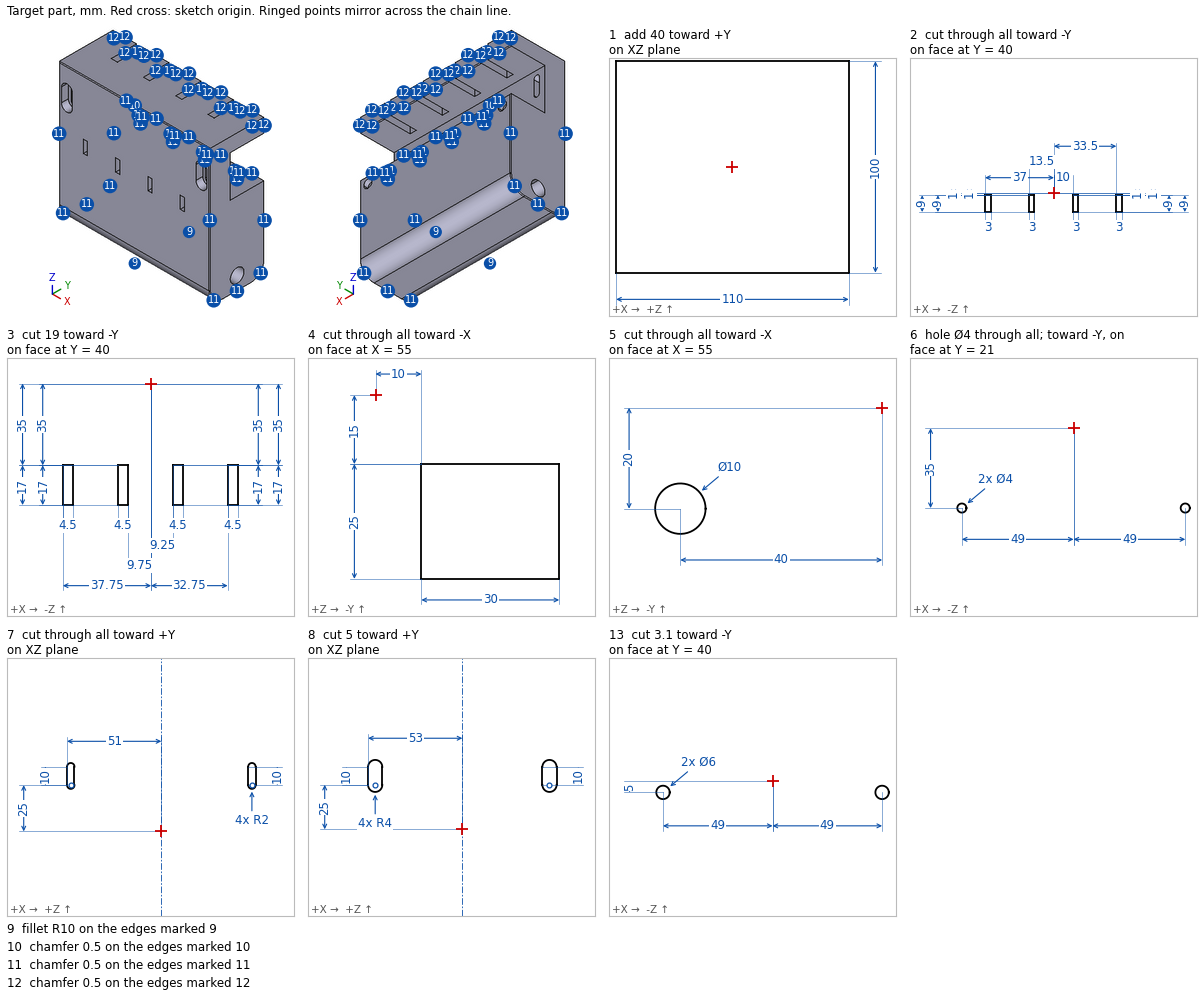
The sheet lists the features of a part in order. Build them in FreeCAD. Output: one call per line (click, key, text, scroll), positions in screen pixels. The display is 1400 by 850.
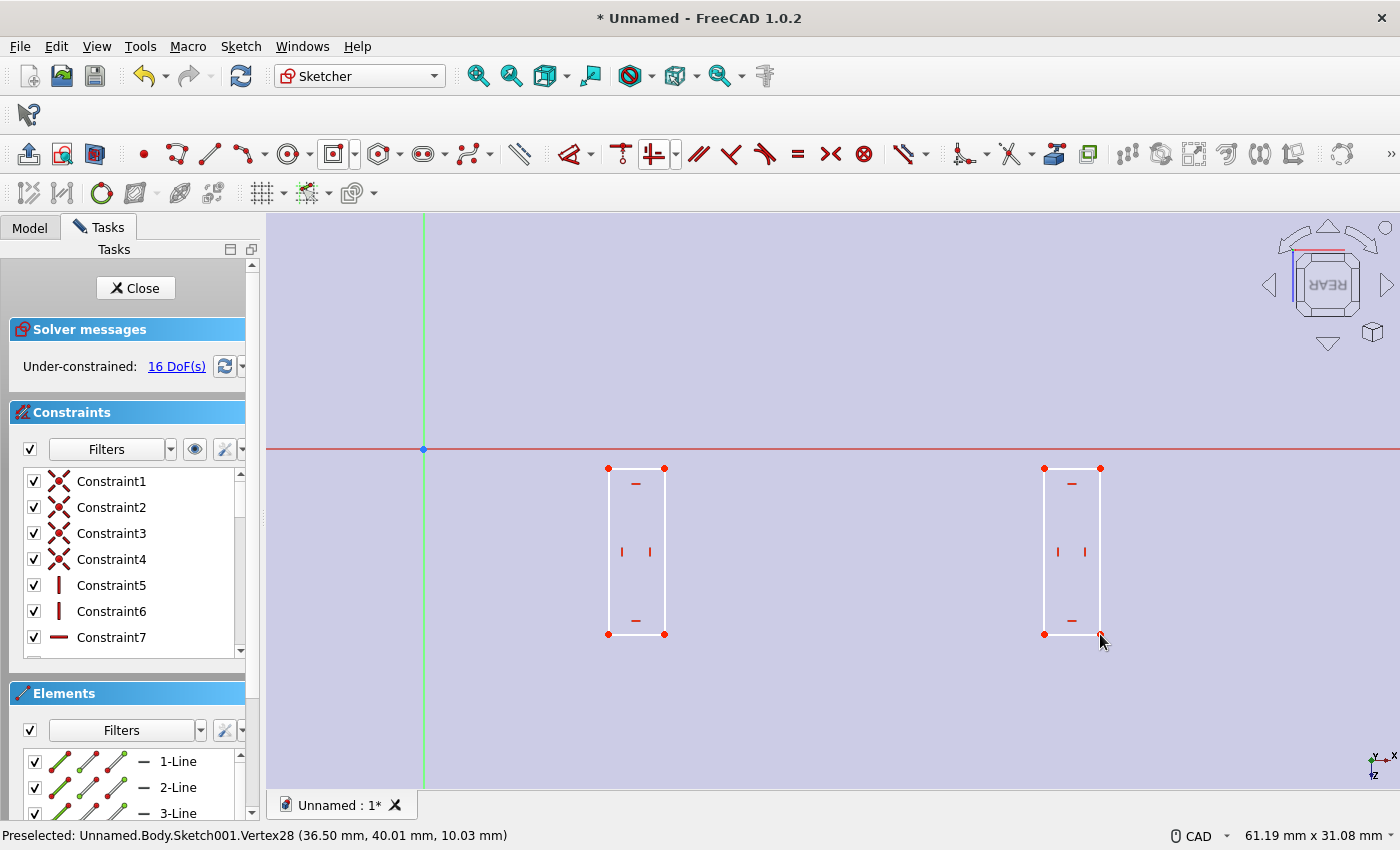
key(d)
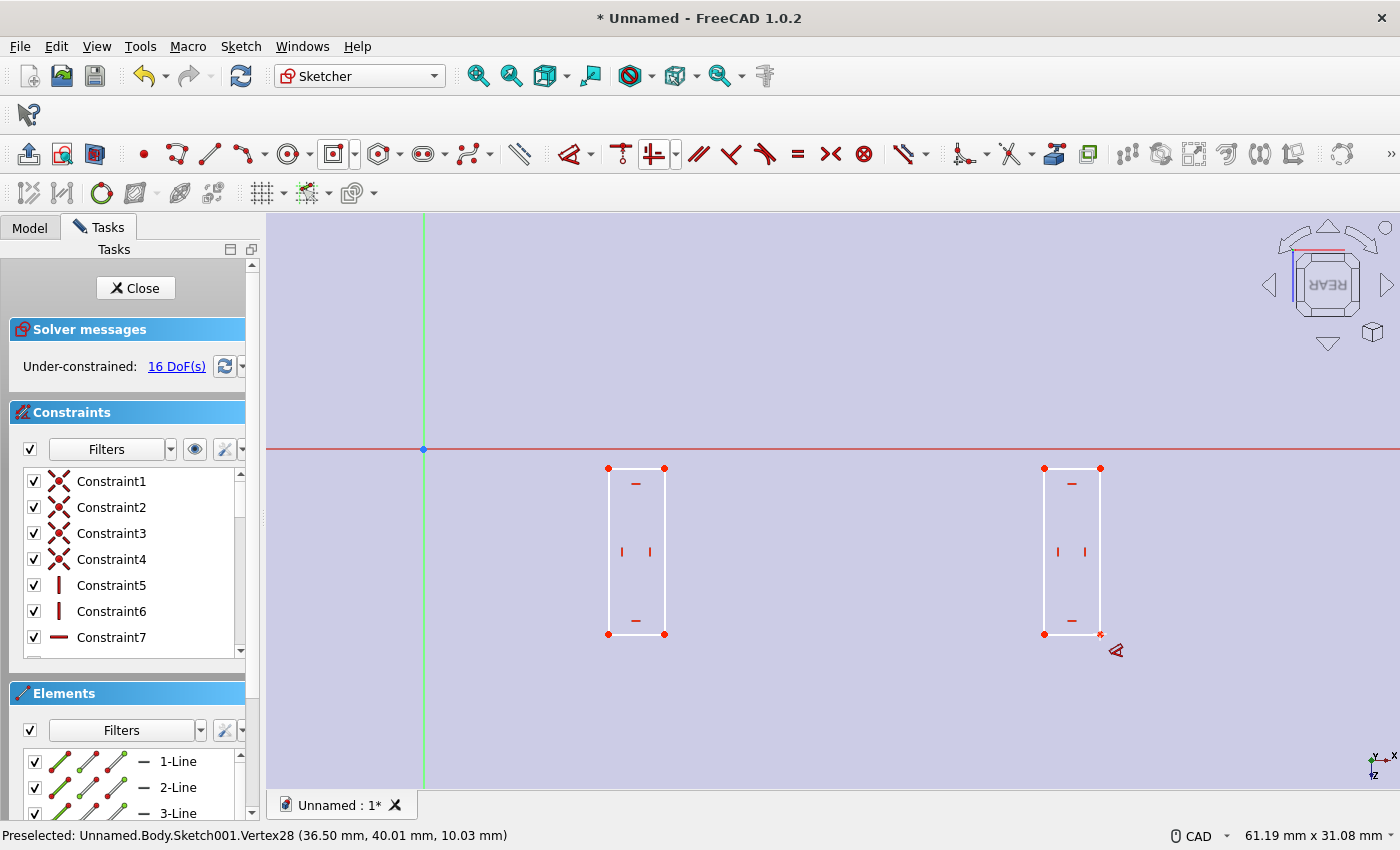
scroll(1046, 468, down, 4)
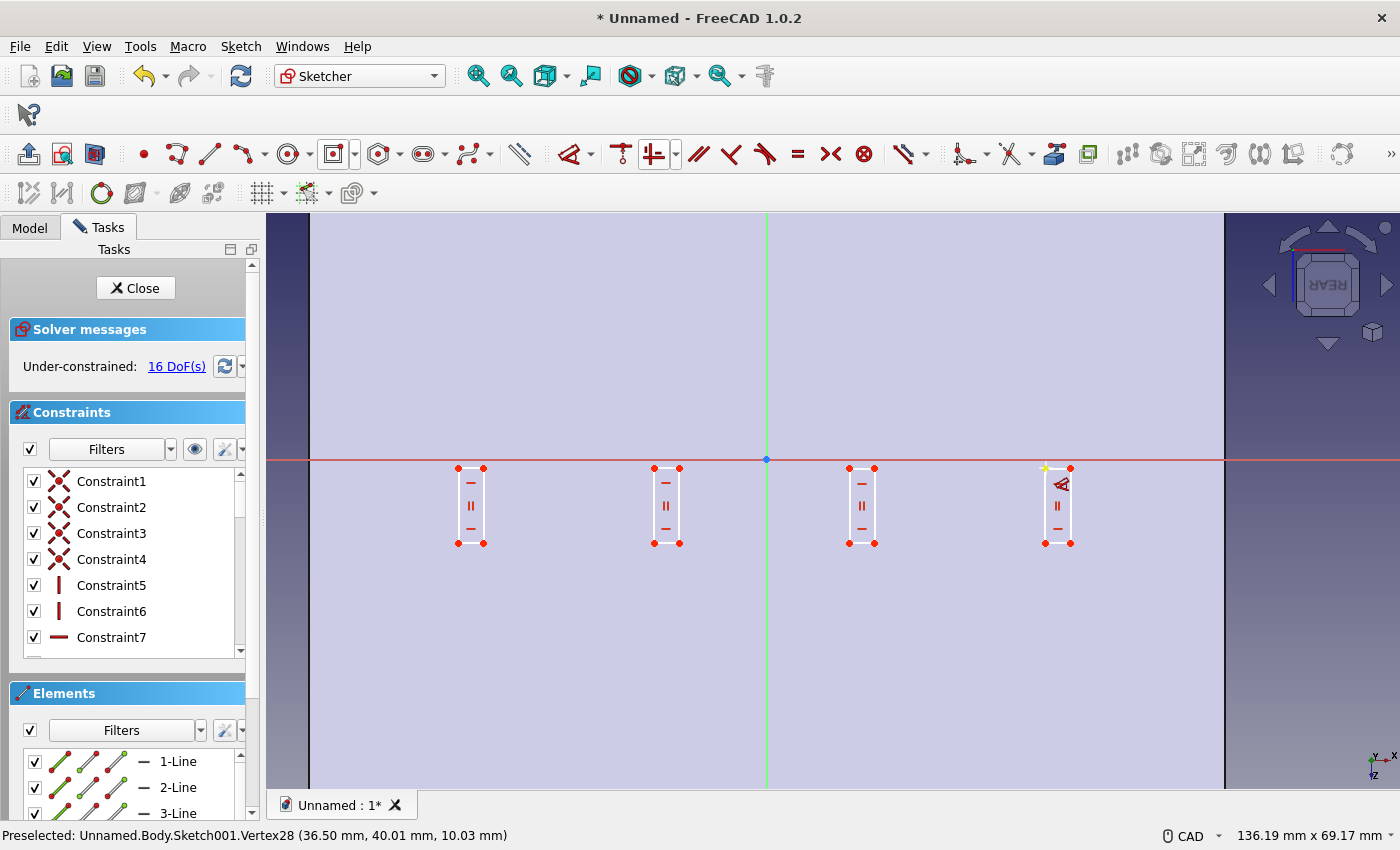
click(459, 491)
click(425, 506)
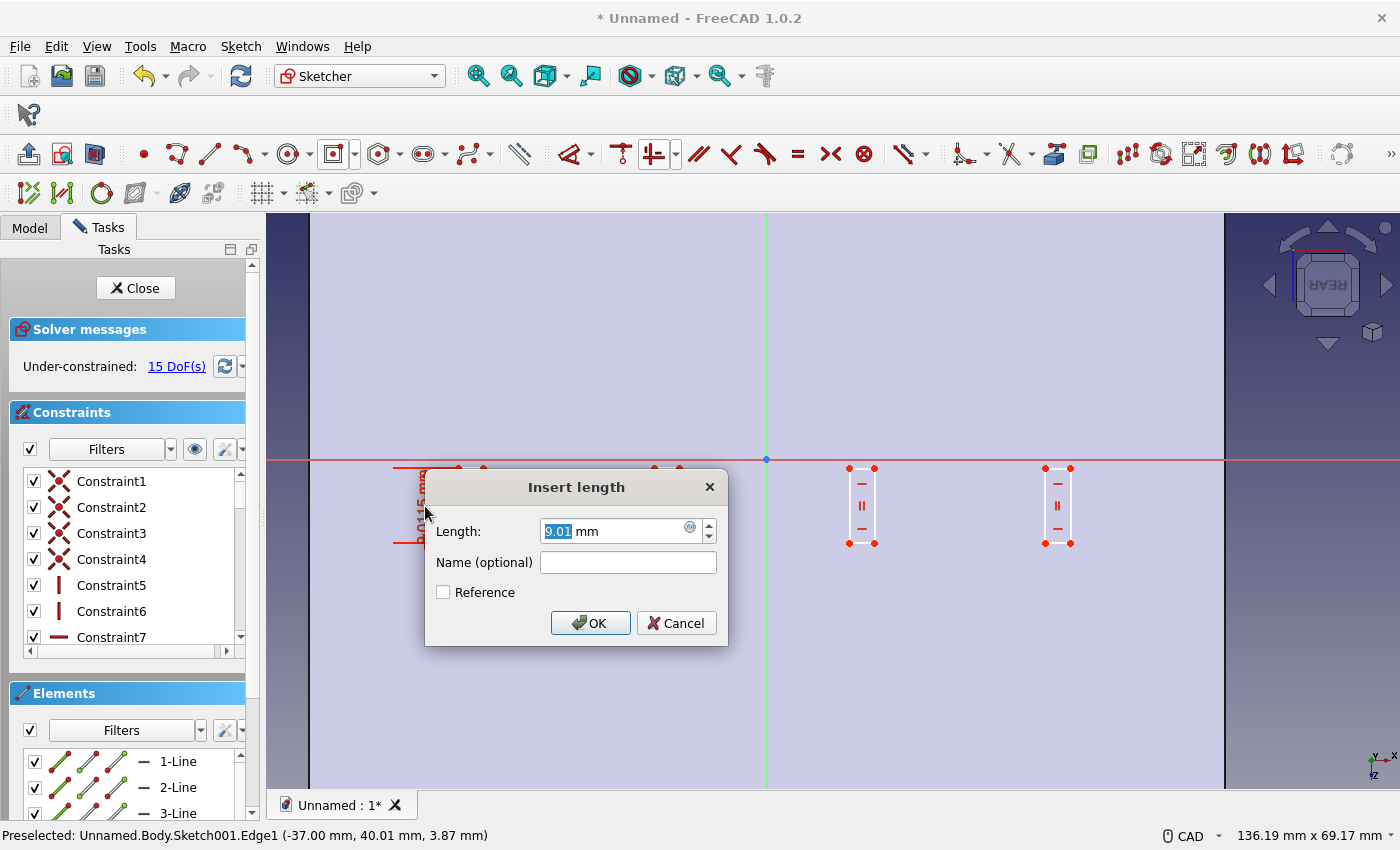
text(9)
key(Return)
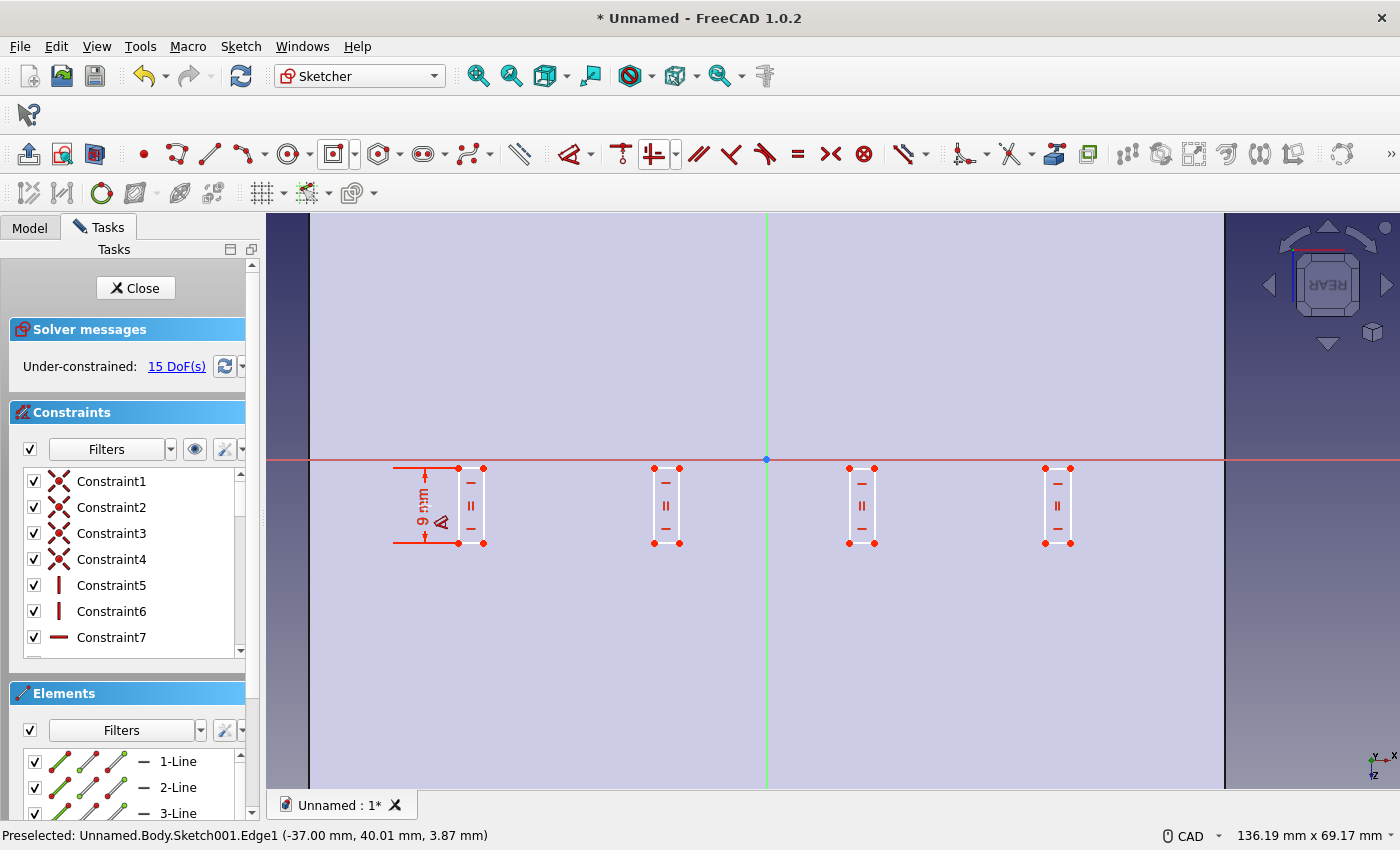
scroll(469, 543, up, 3)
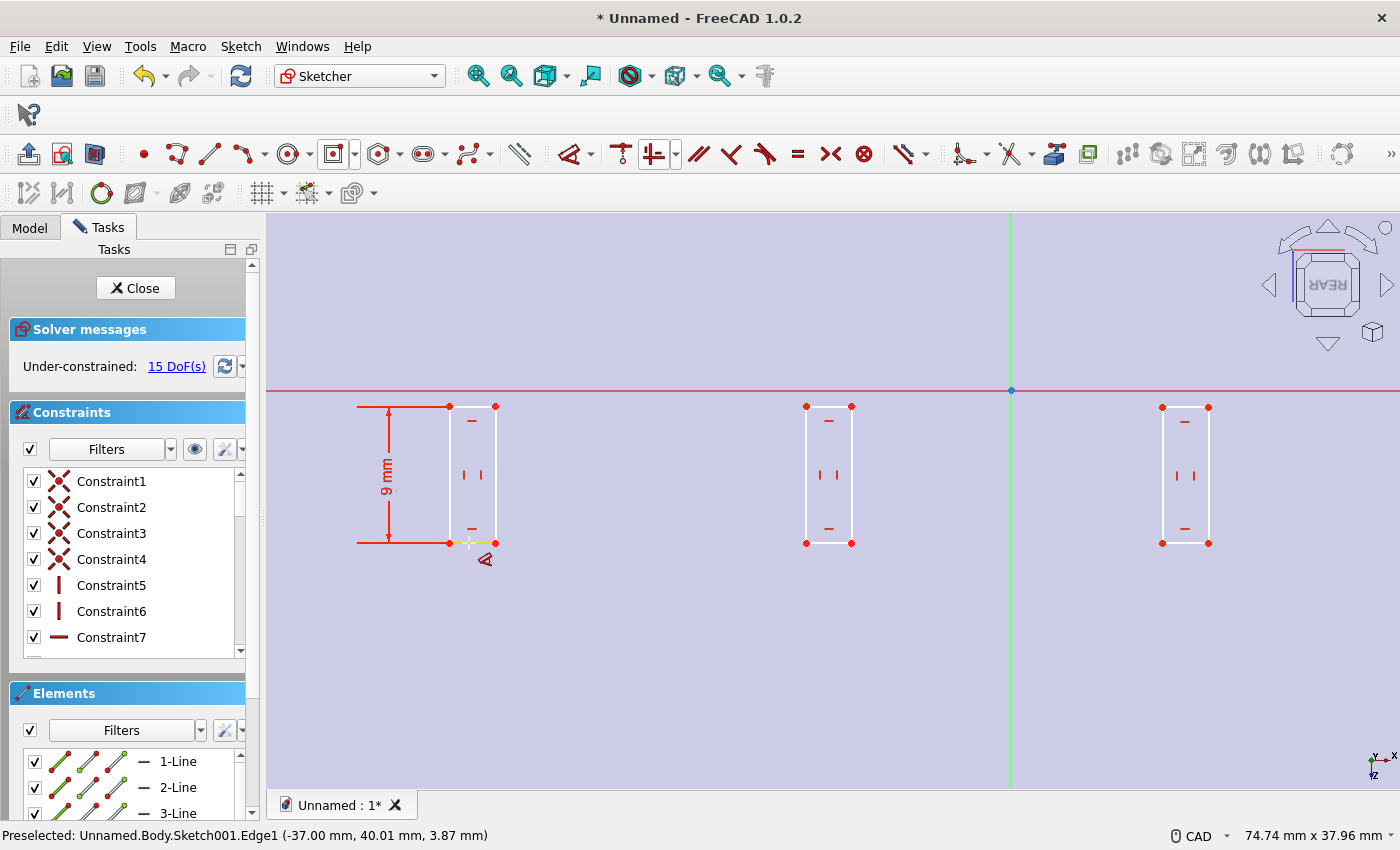
click(468, 543)
click(473, 577)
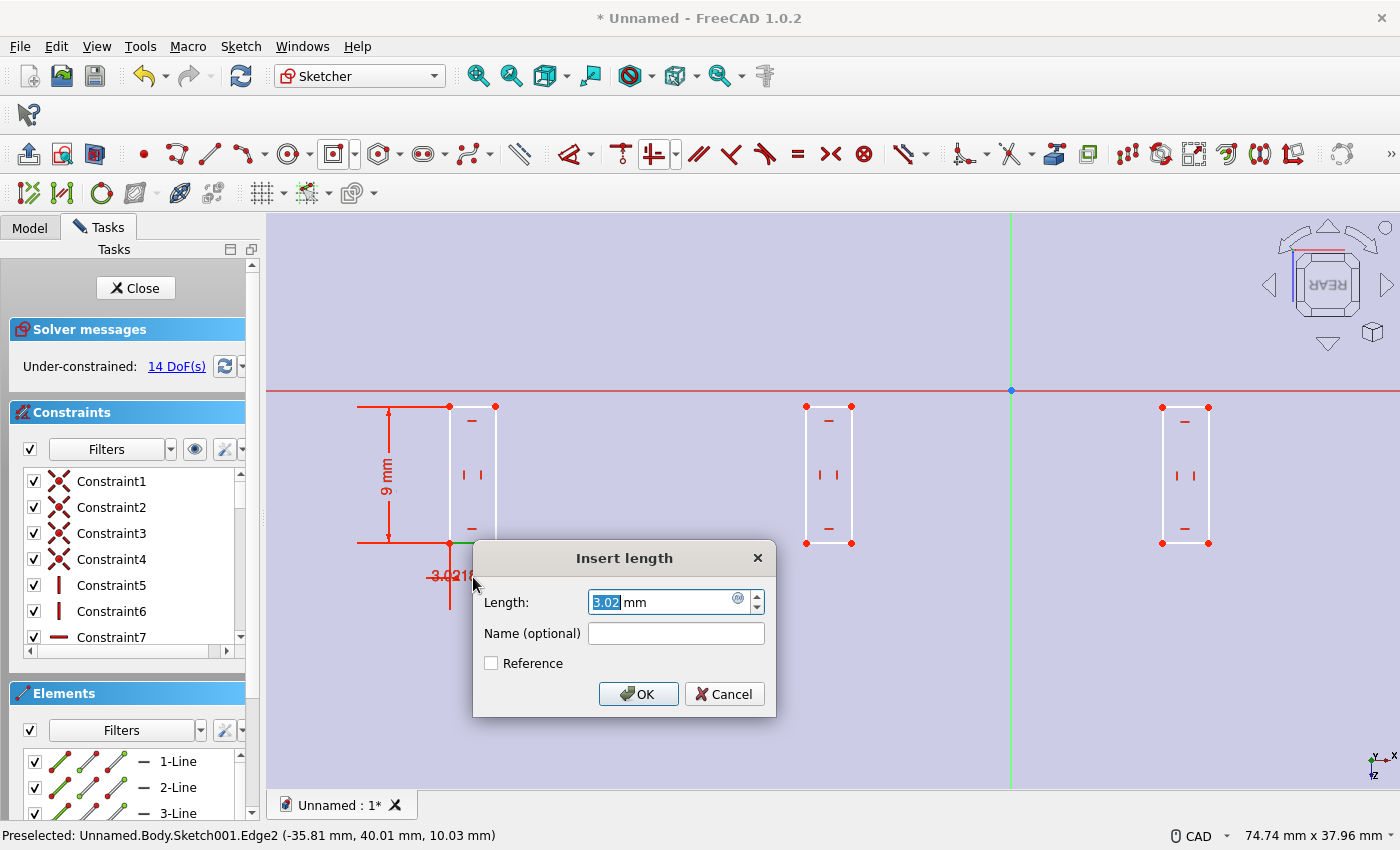
text(3)
key(Return)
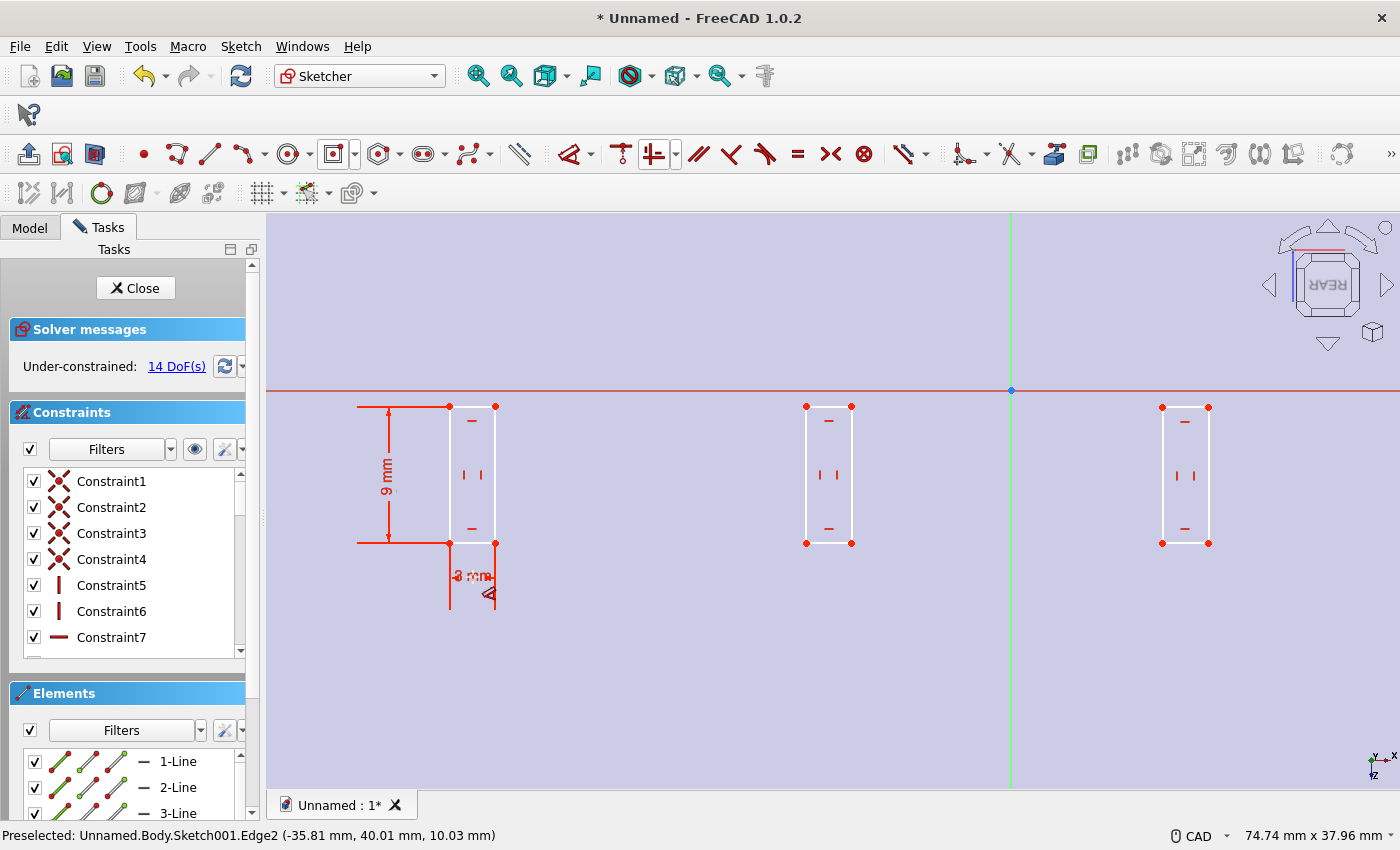
click(806, 448)
click(772, 475)